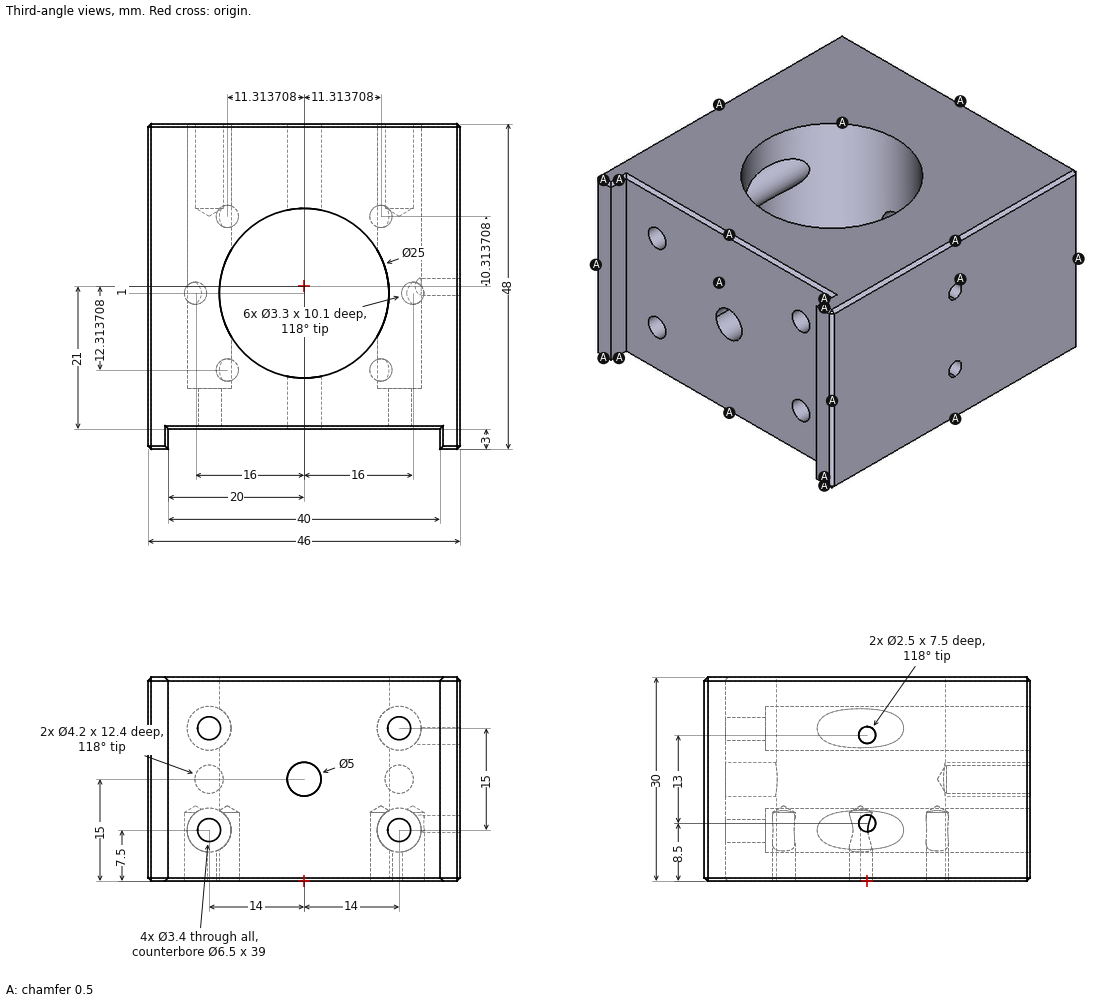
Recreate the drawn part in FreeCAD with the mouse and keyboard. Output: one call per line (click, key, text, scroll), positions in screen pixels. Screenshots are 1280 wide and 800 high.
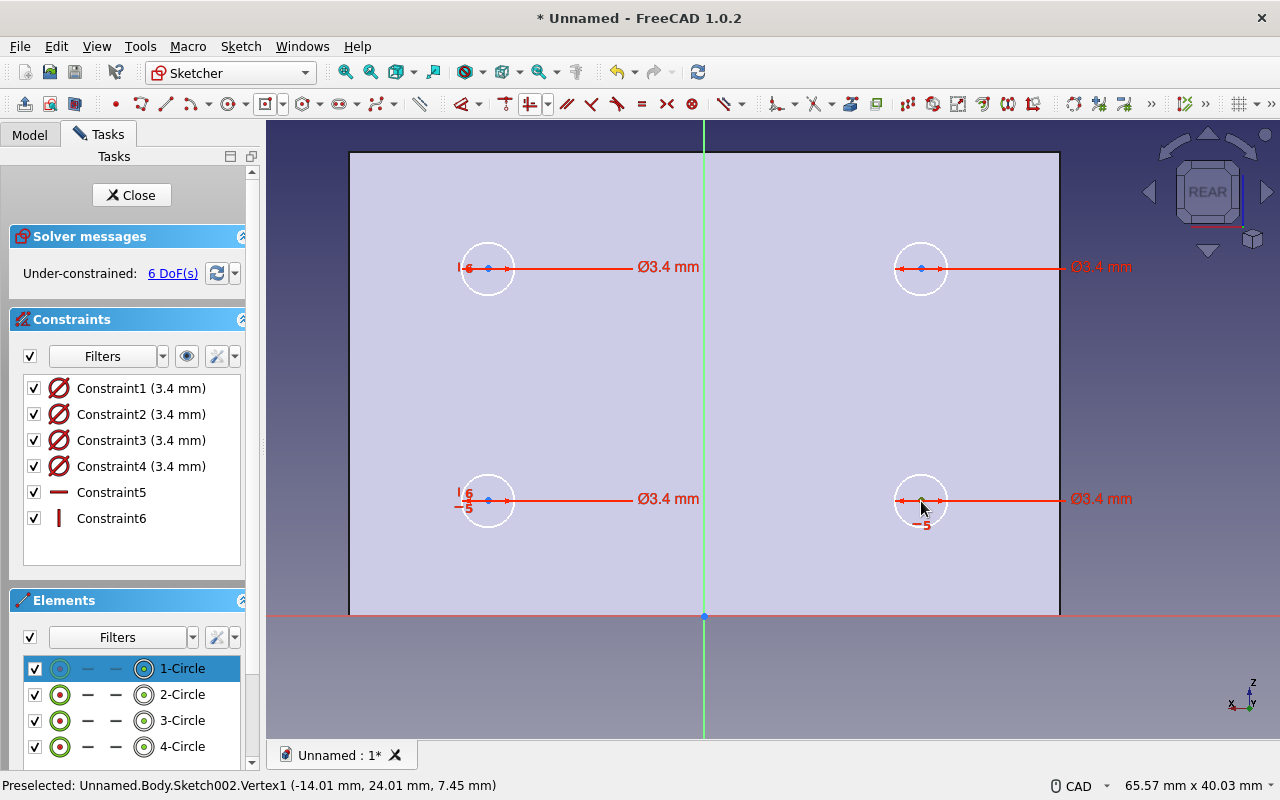
click(921, 269)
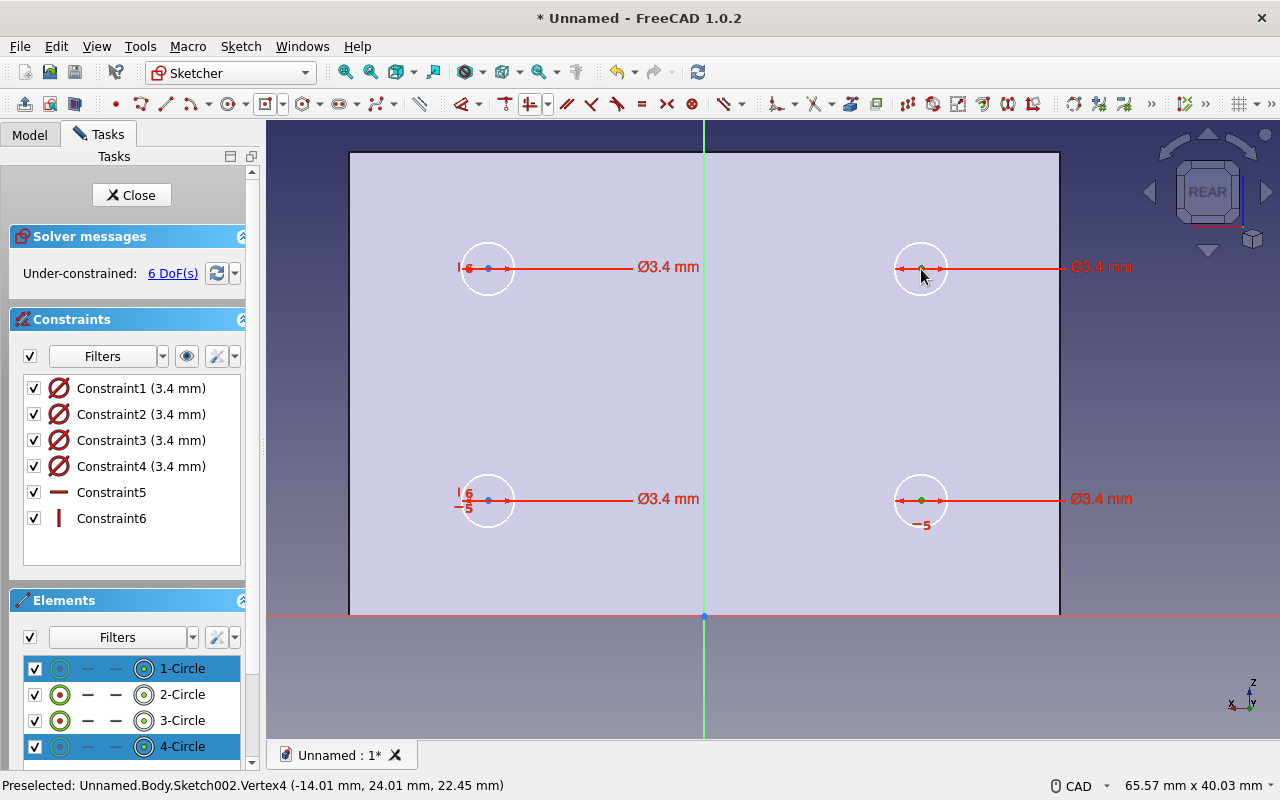
key(v)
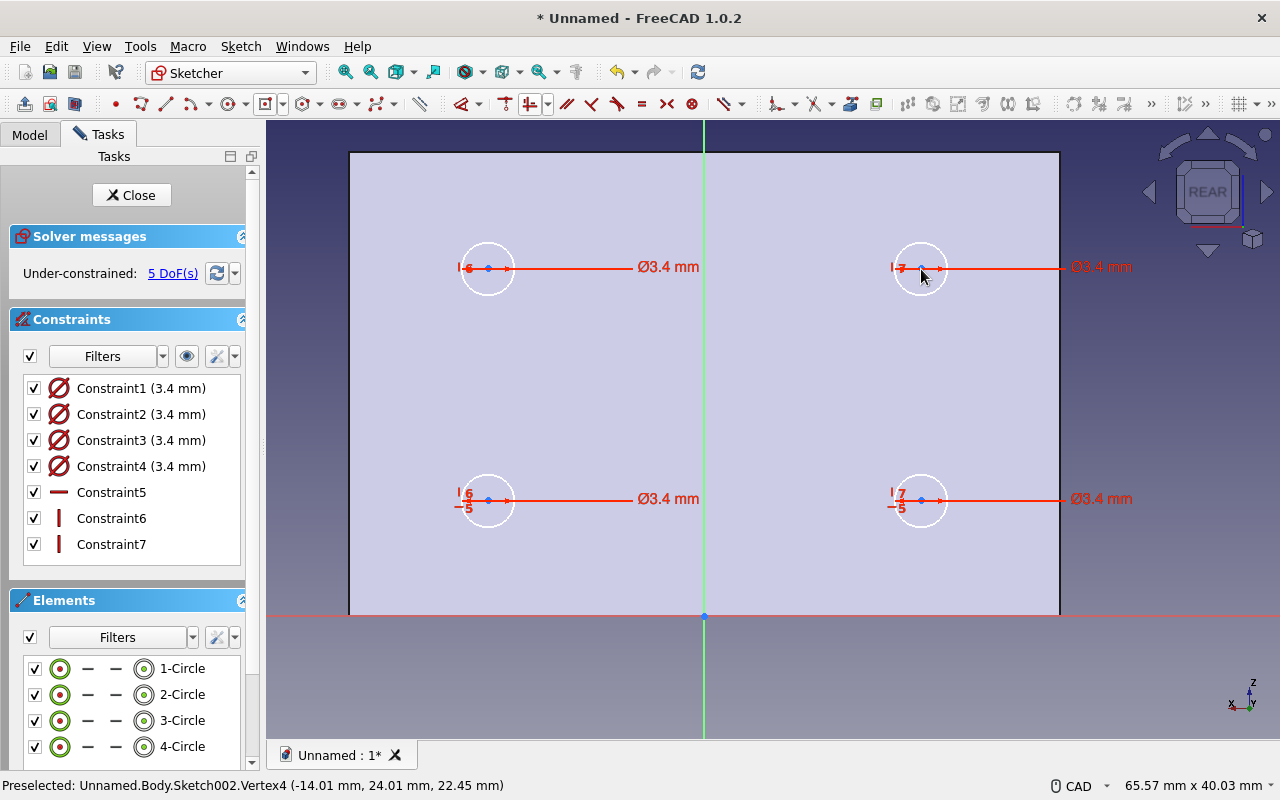
click(488, 269)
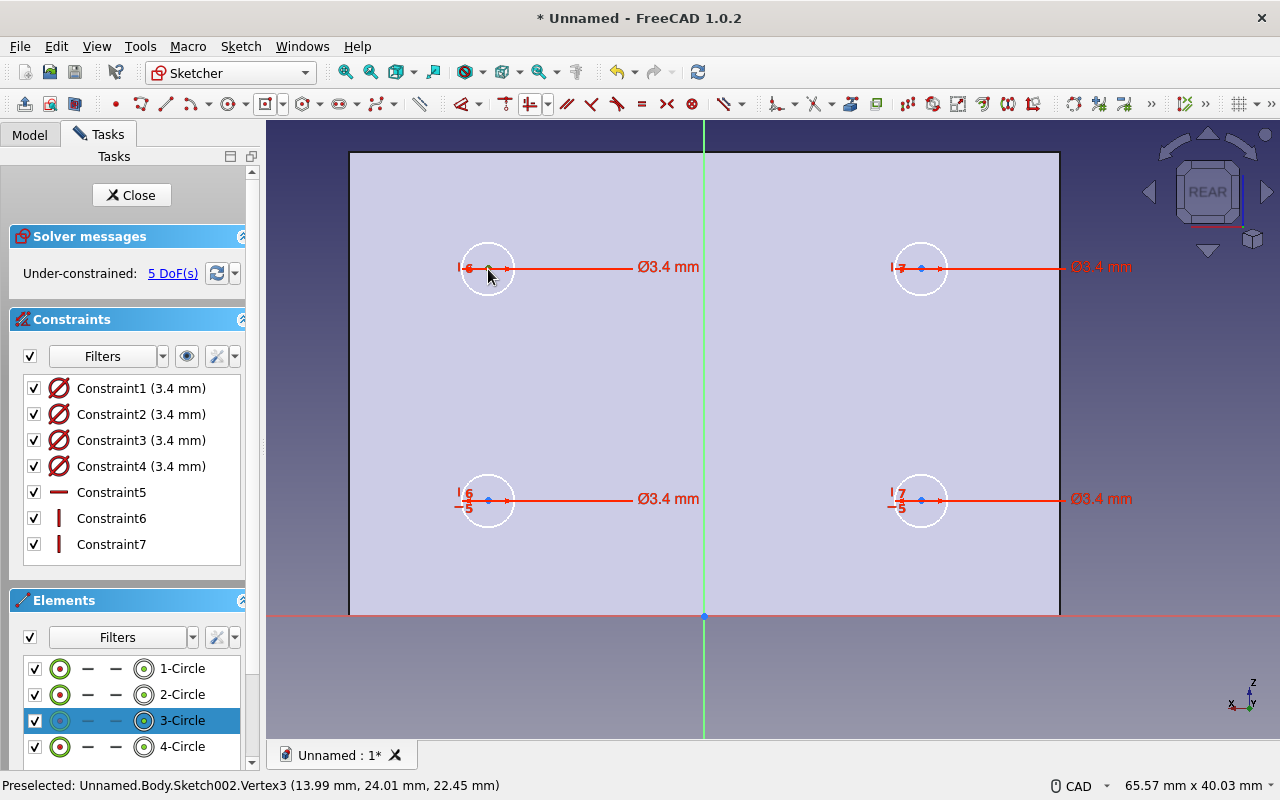
click(921, 269)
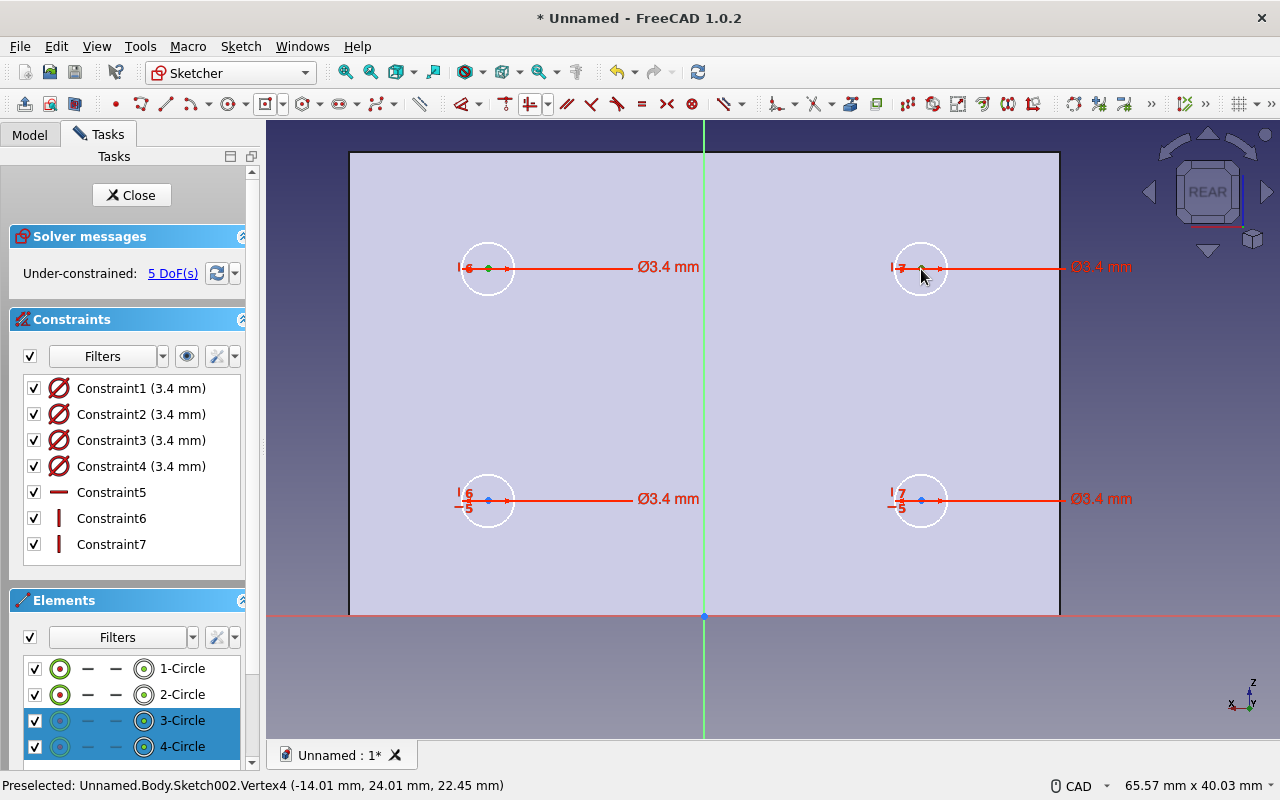
click(548, 104)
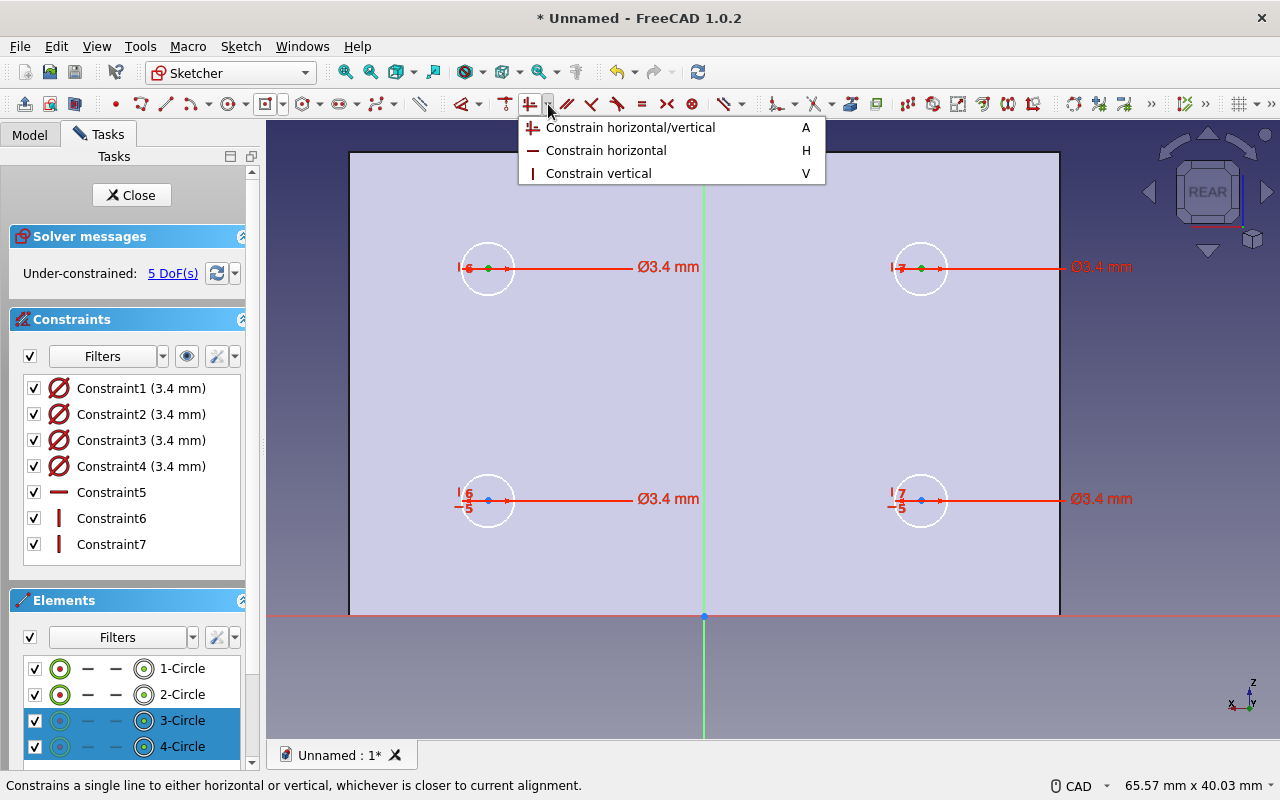
click(672, 150)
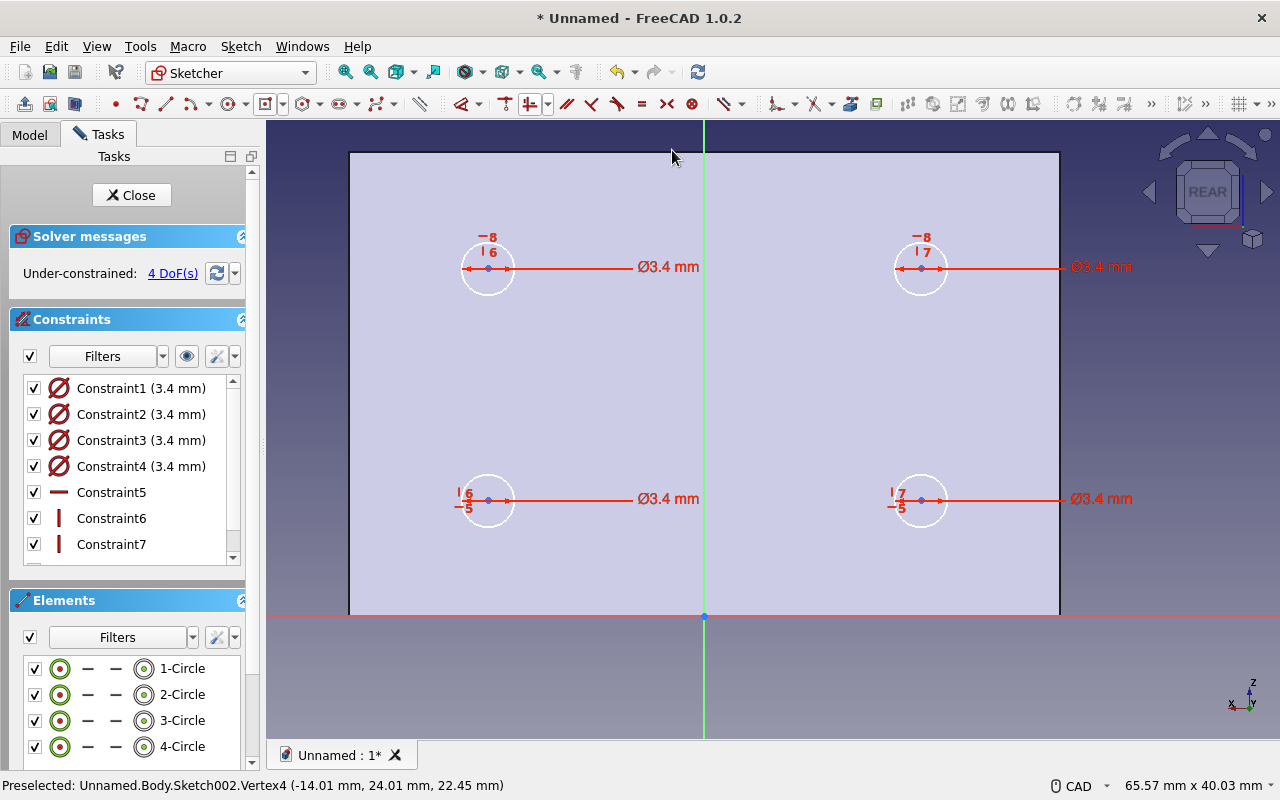
click(460, 104)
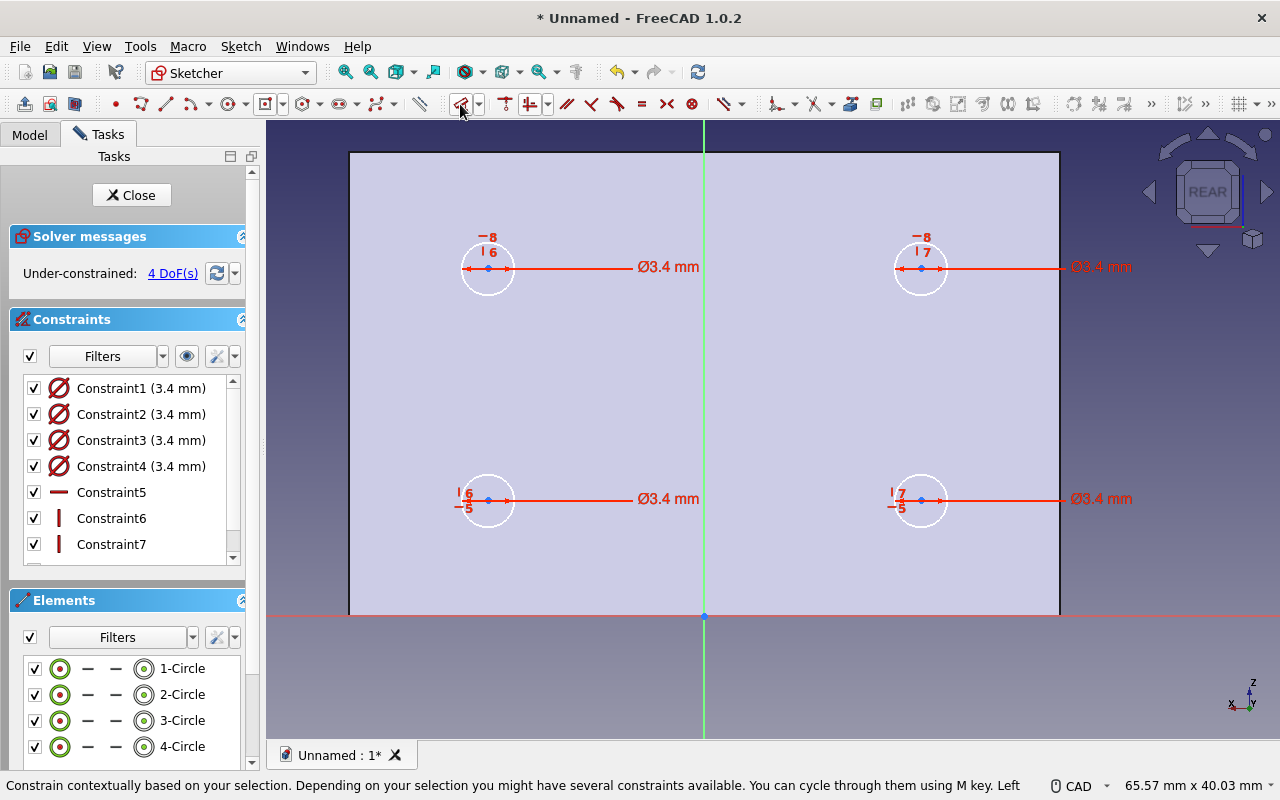
click(921, 501)
click(813, 650)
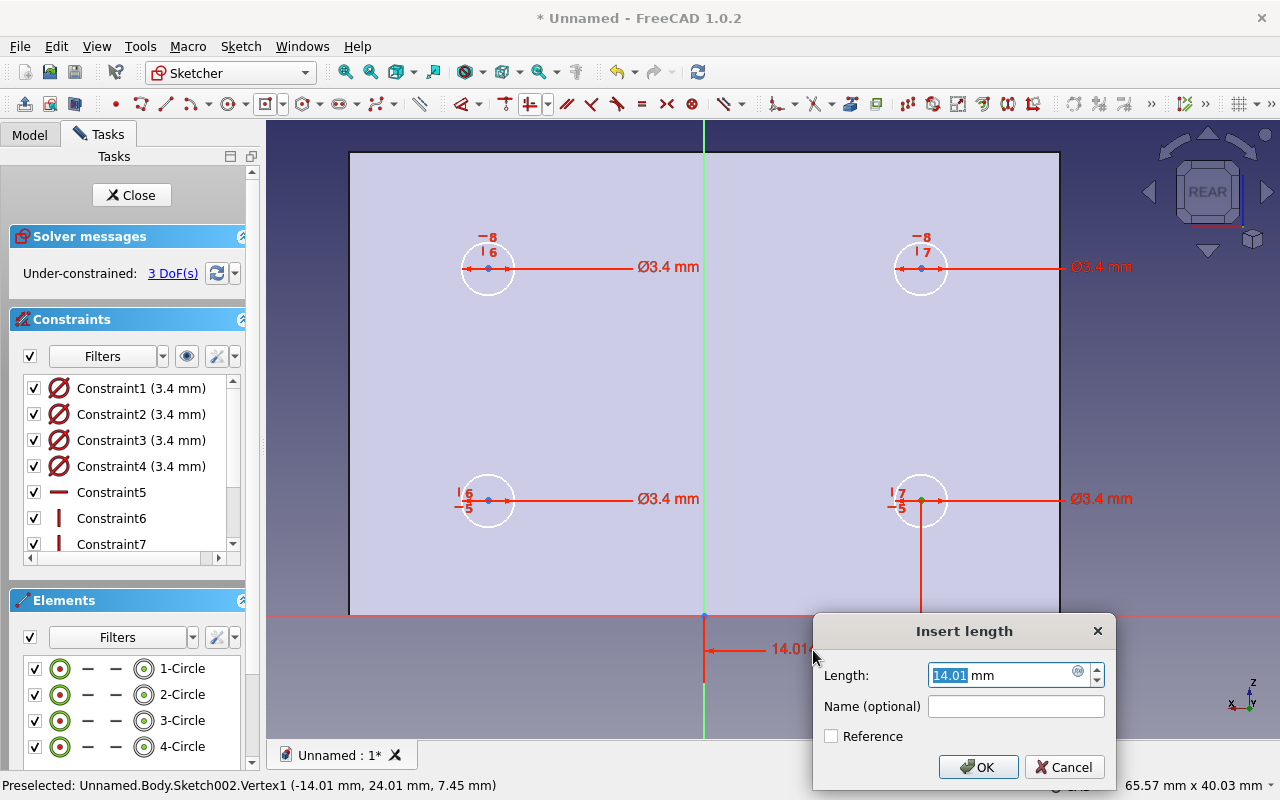
text(14)
key(Return)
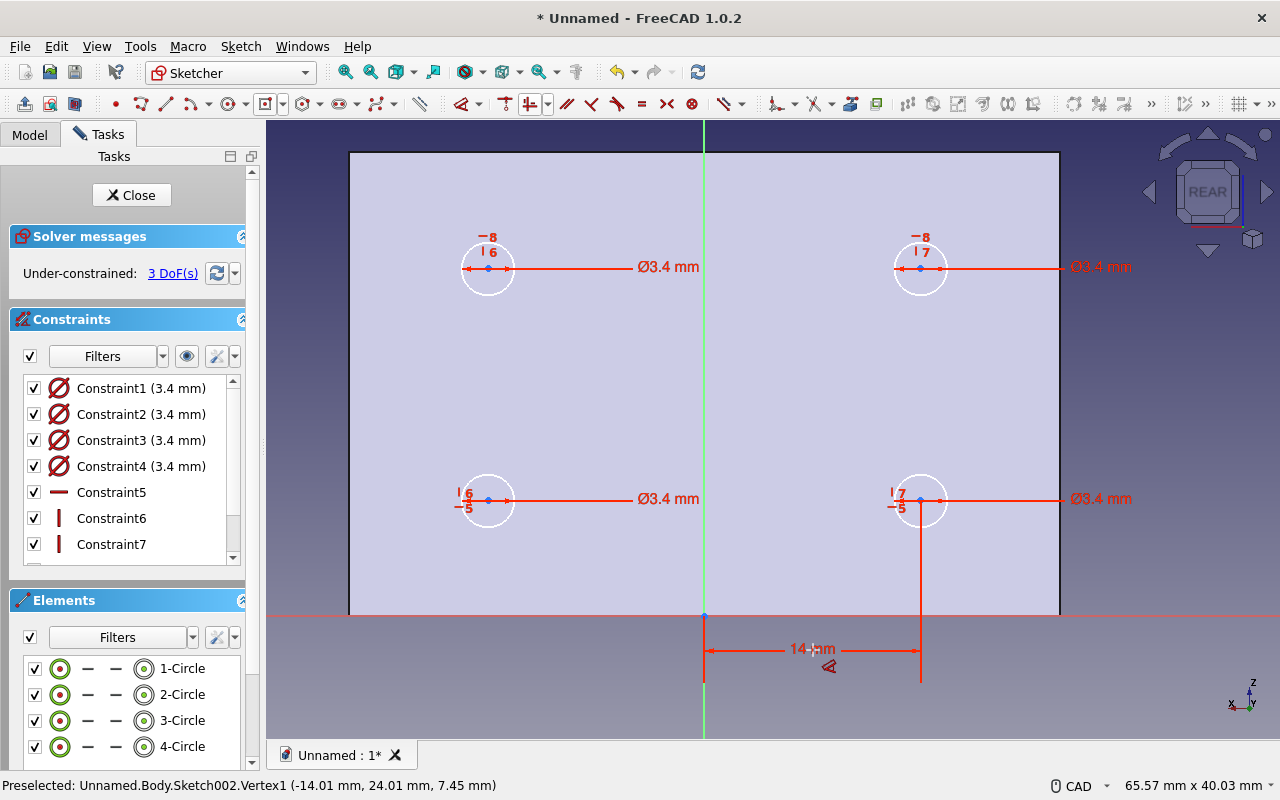
click(488, 501)
click(596, 650)